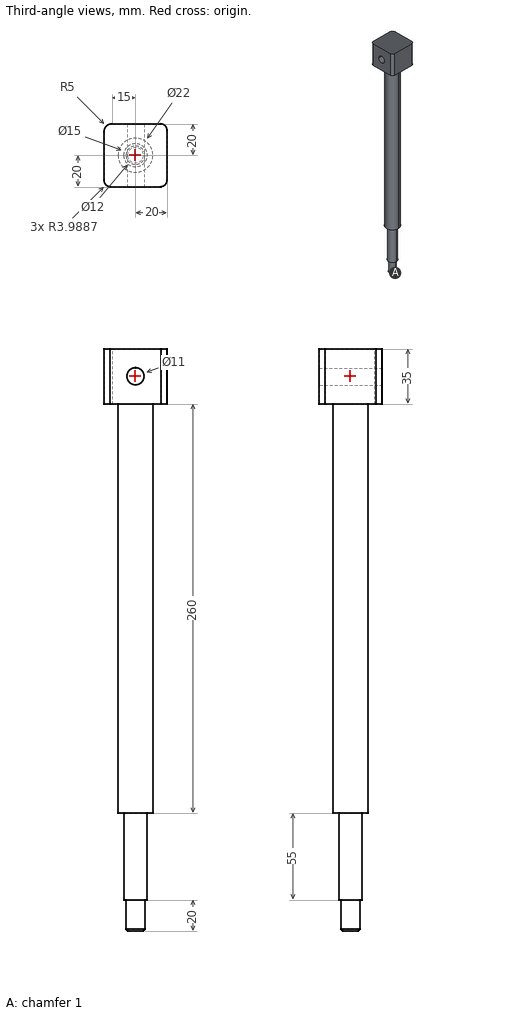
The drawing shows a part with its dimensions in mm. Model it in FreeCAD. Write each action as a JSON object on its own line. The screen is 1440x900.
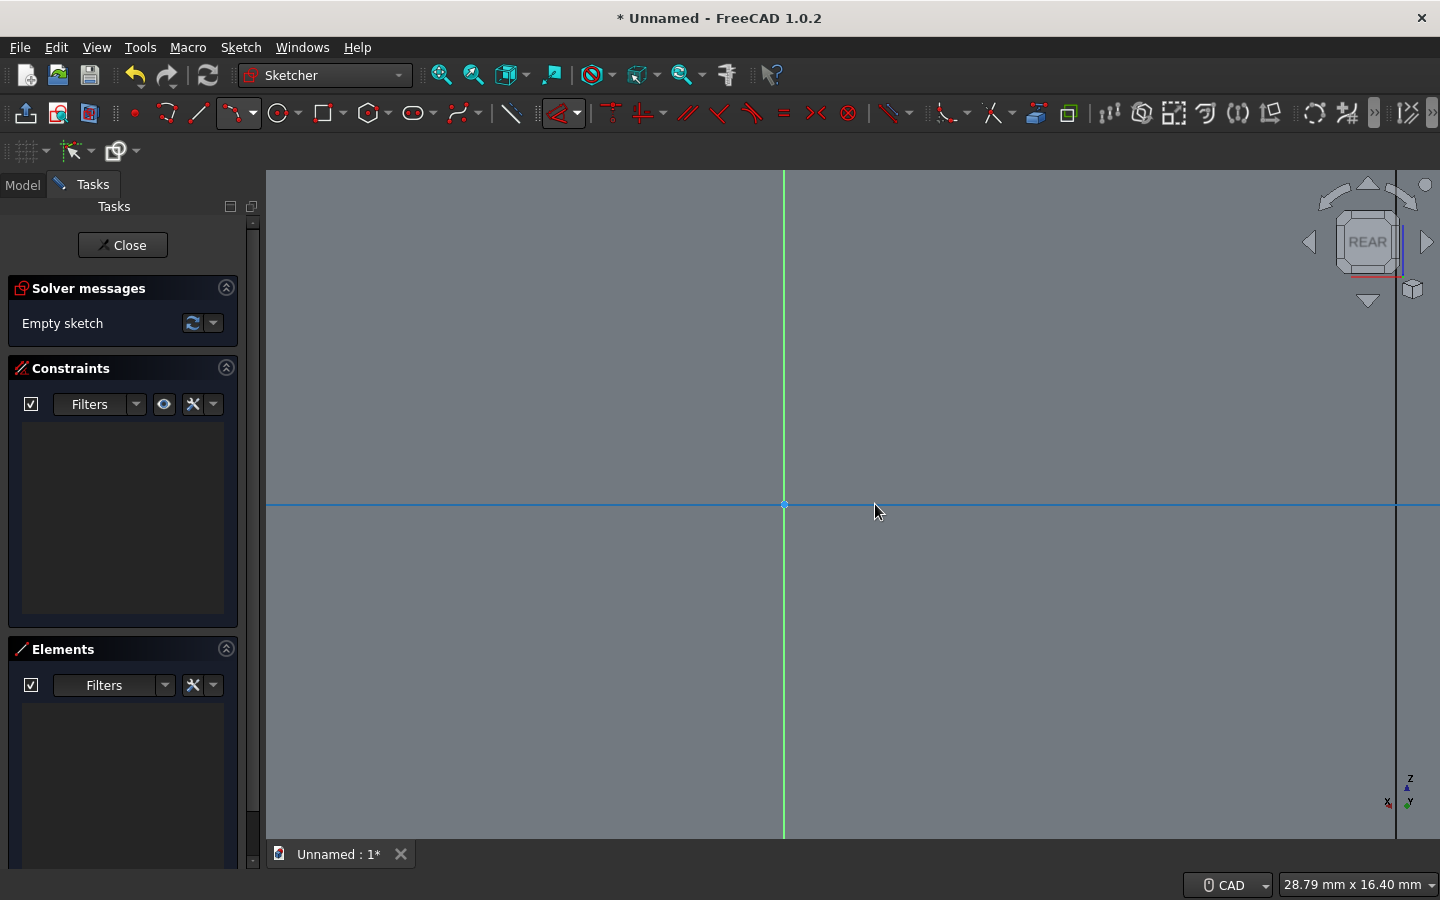
{"action": "left_click", "coordinate": [278, 114]}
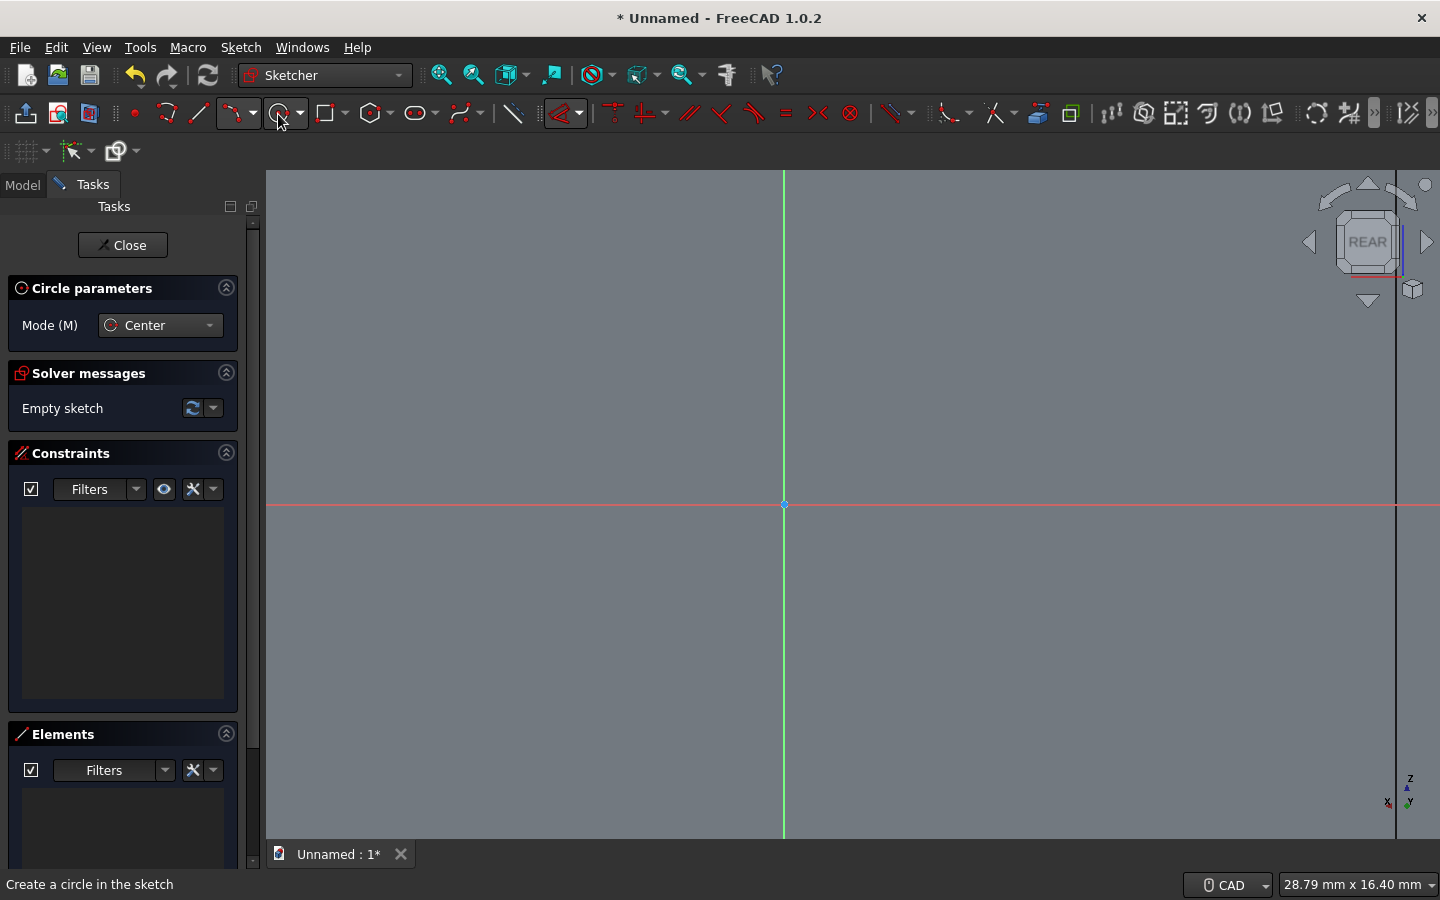
{"action": "left_click", "coordinate": [784, 504]}
{"action": "left_click", "coordinate": [943, 346]}
{"action": "key", "text": "Escape"}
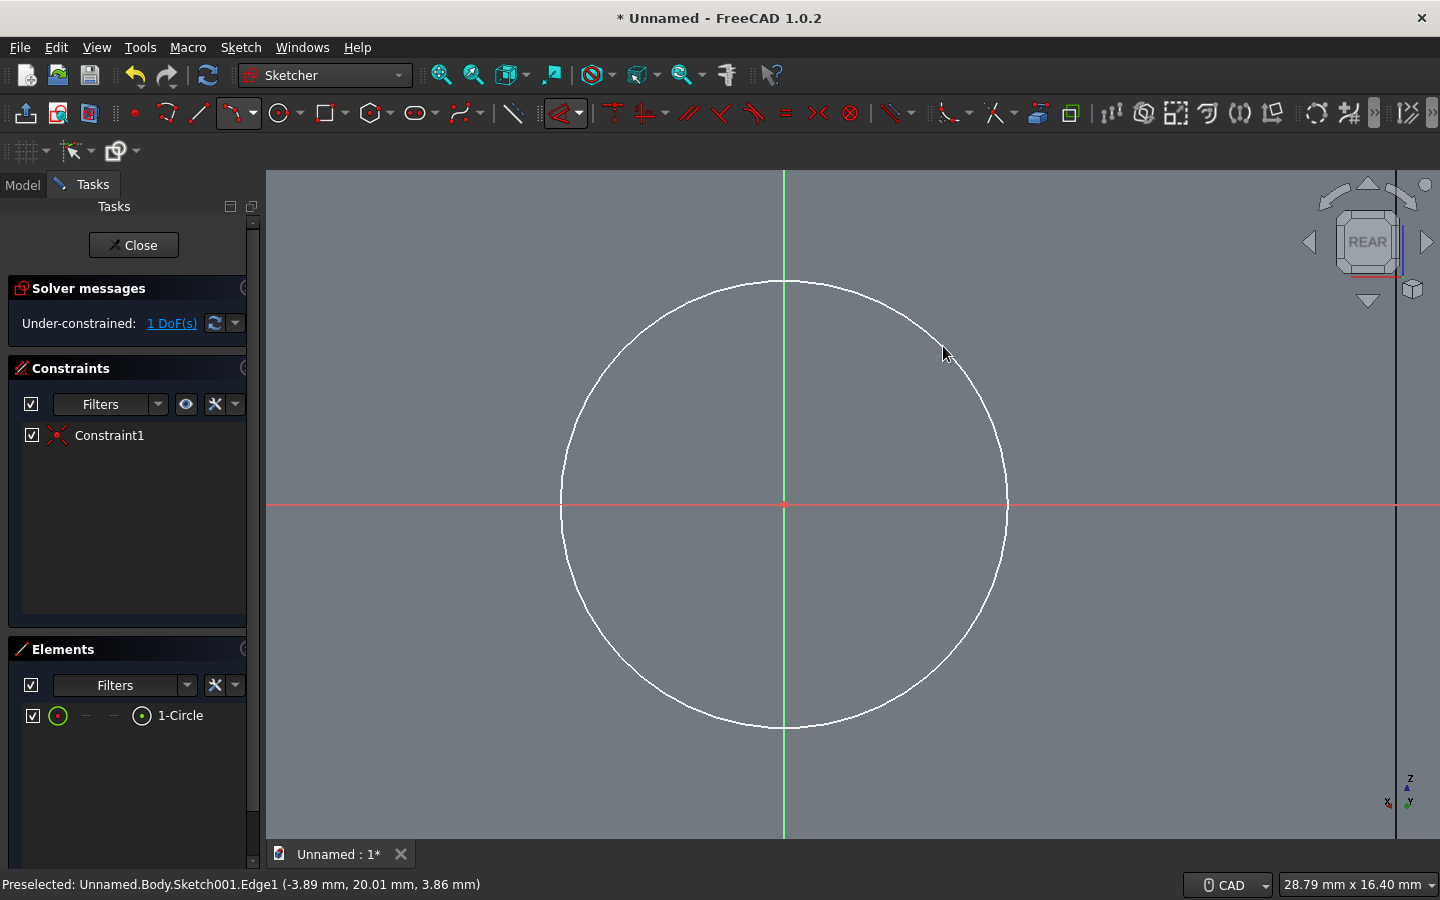
{"action": "left_click", "coordinate": [942, 346]}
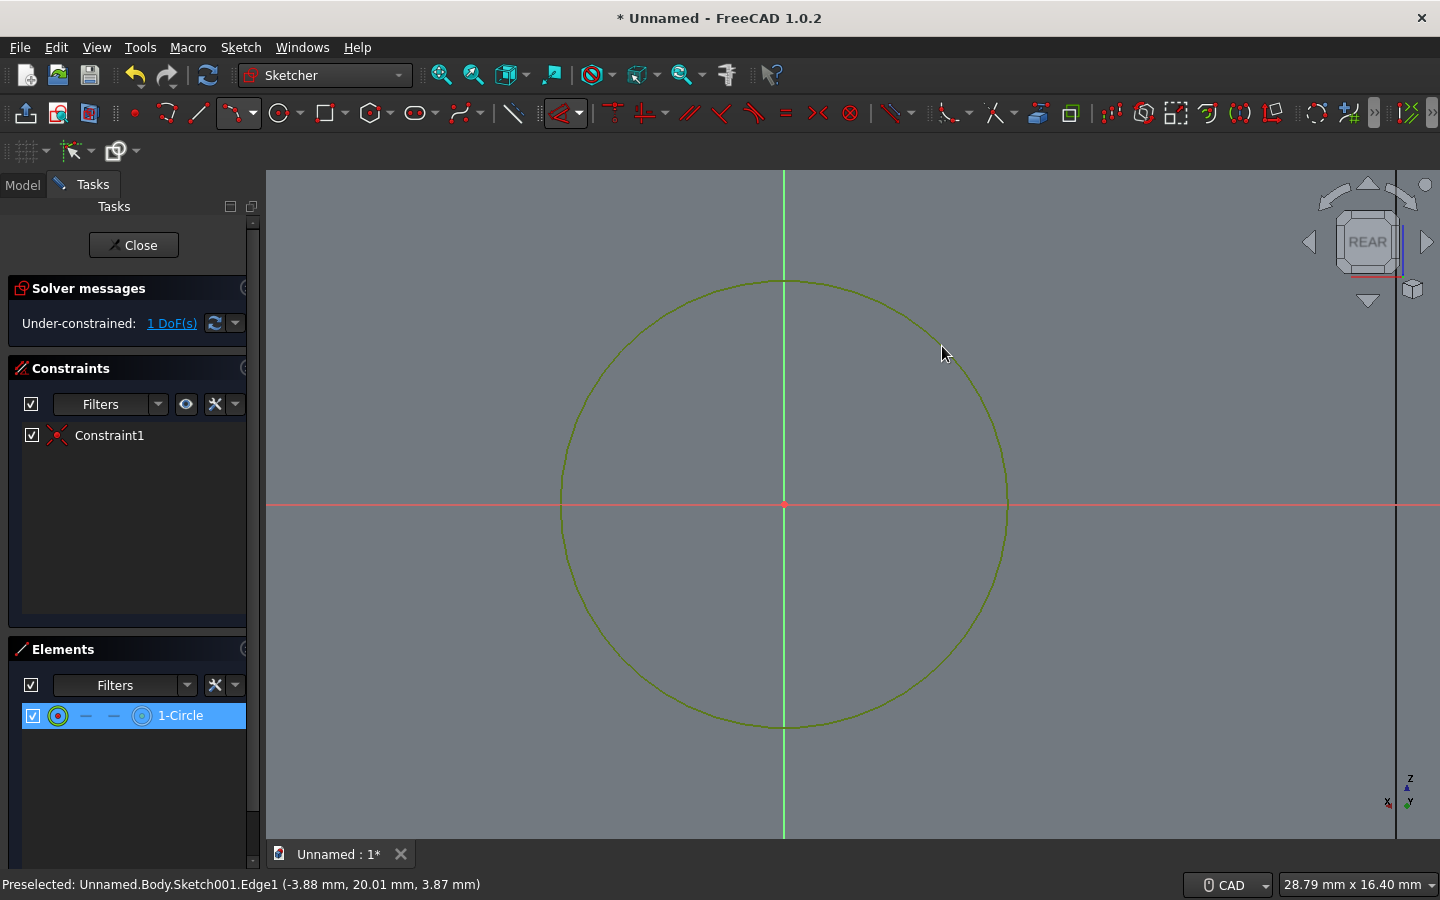
{"action": "left_click", "coordinate": [582, 114]}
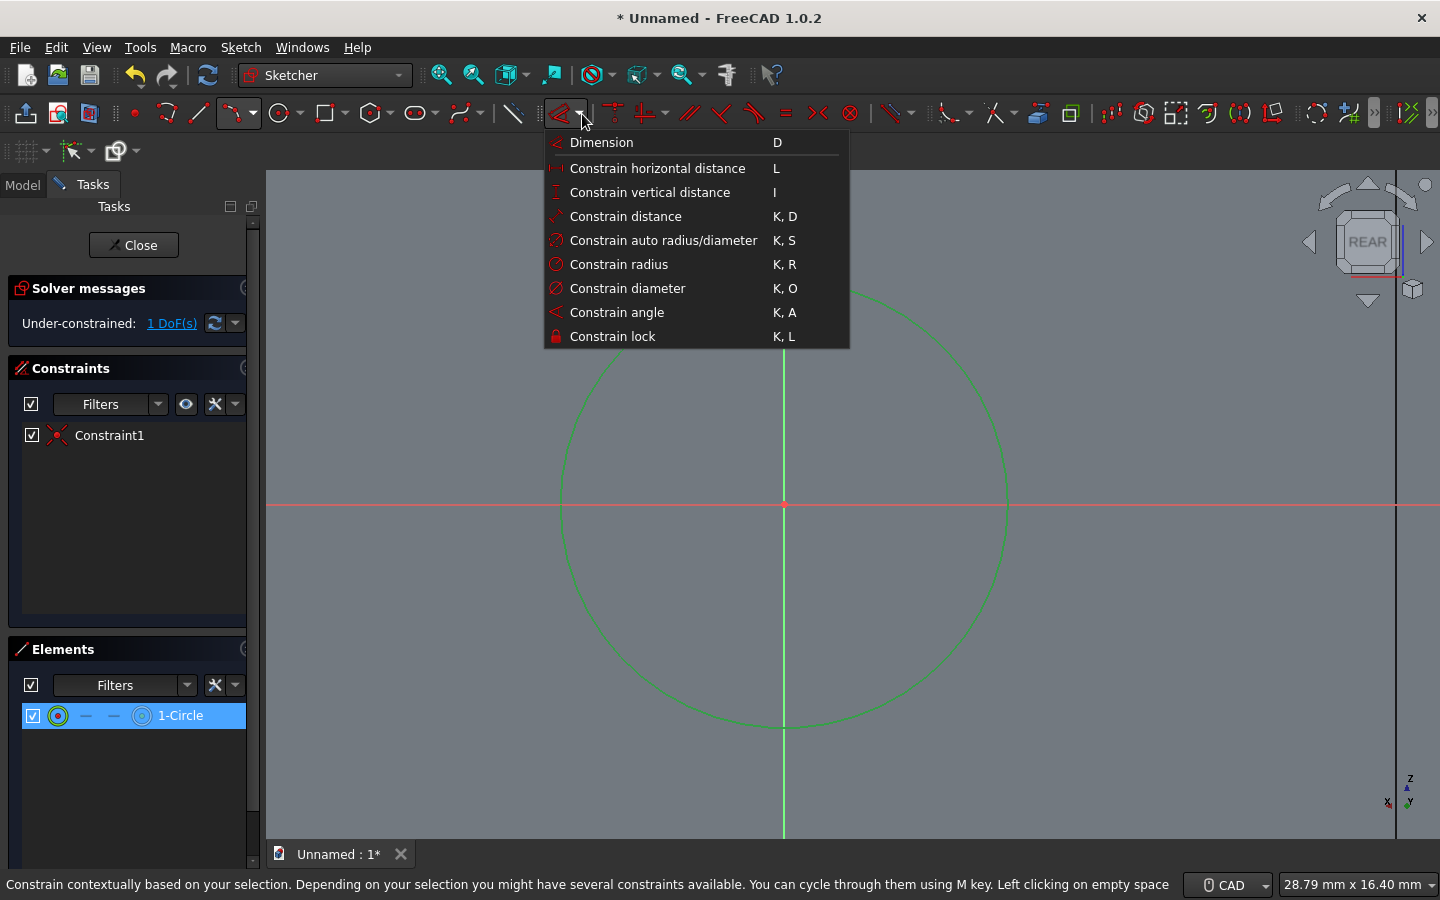
{"action": "left_click", "coordinate": [697, 288]}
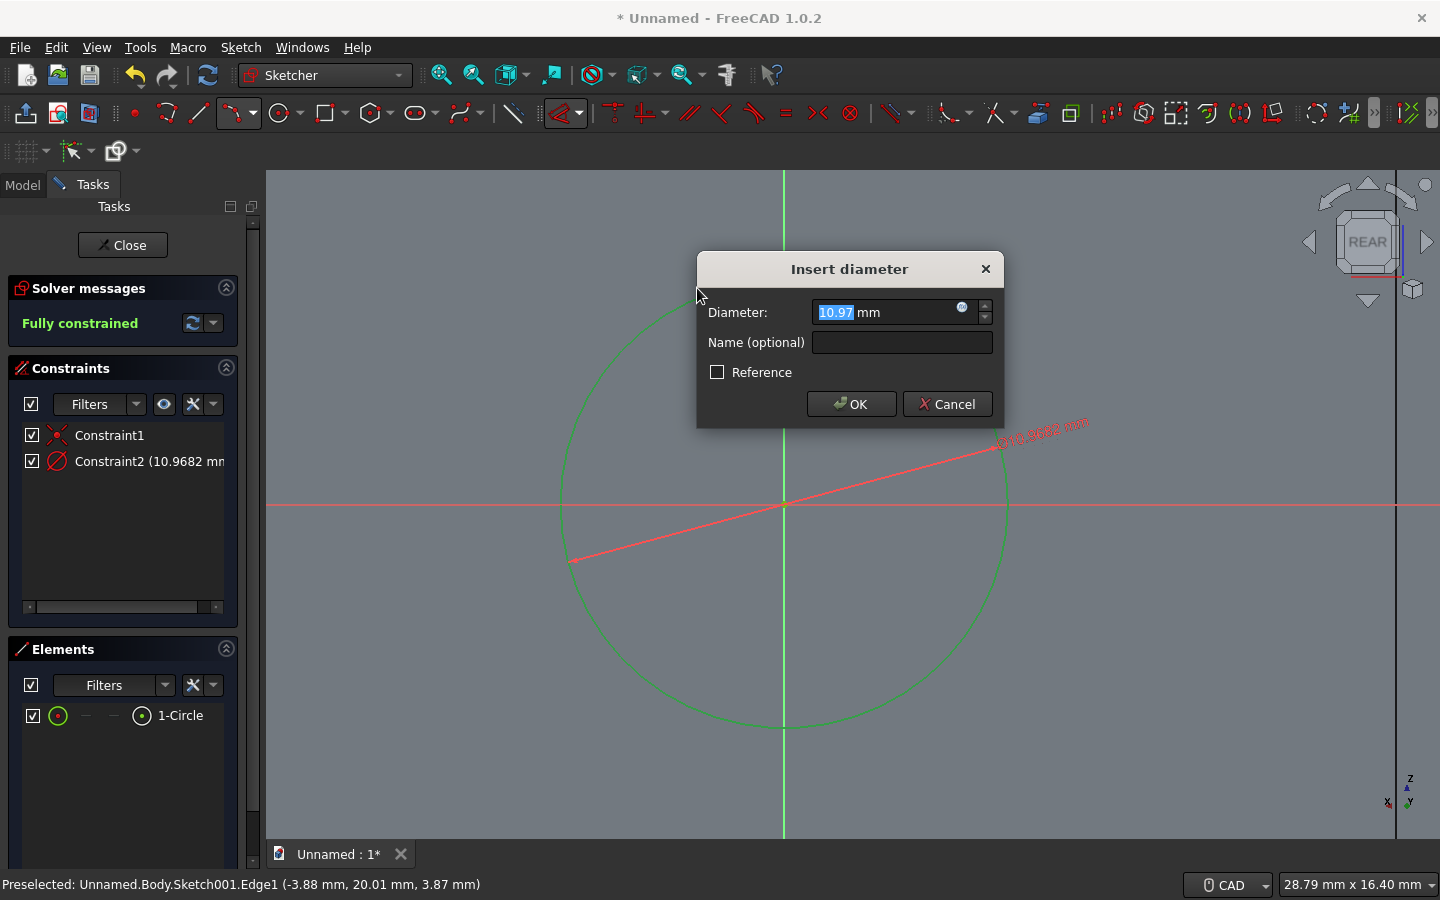
{"action": "type", "text": "11"}
{"action": "key", "text": "Return"}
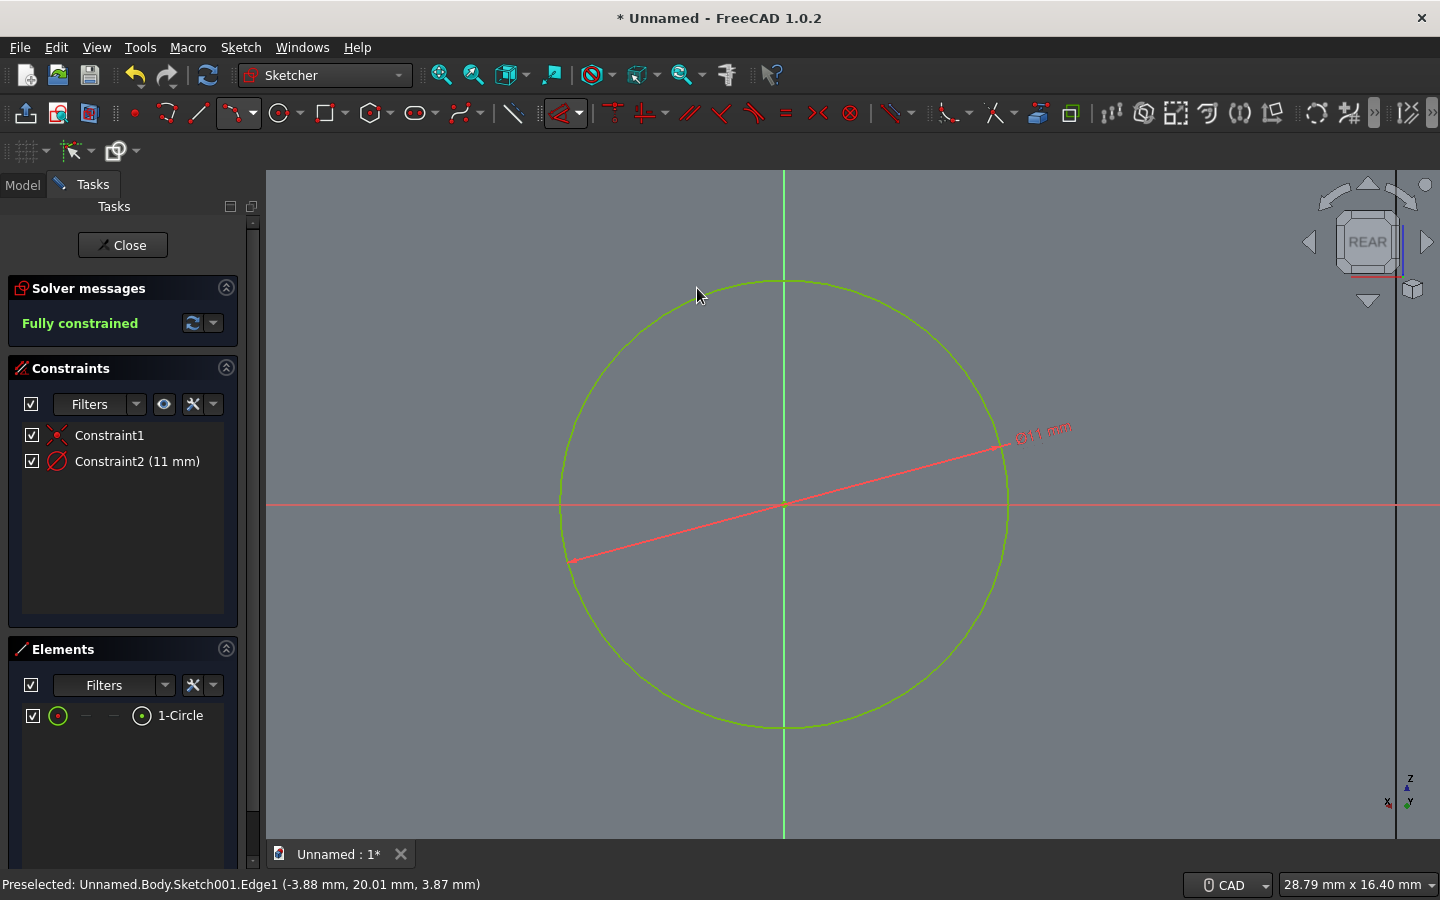
{"action": "left_click", "coordinate": [123, 245]}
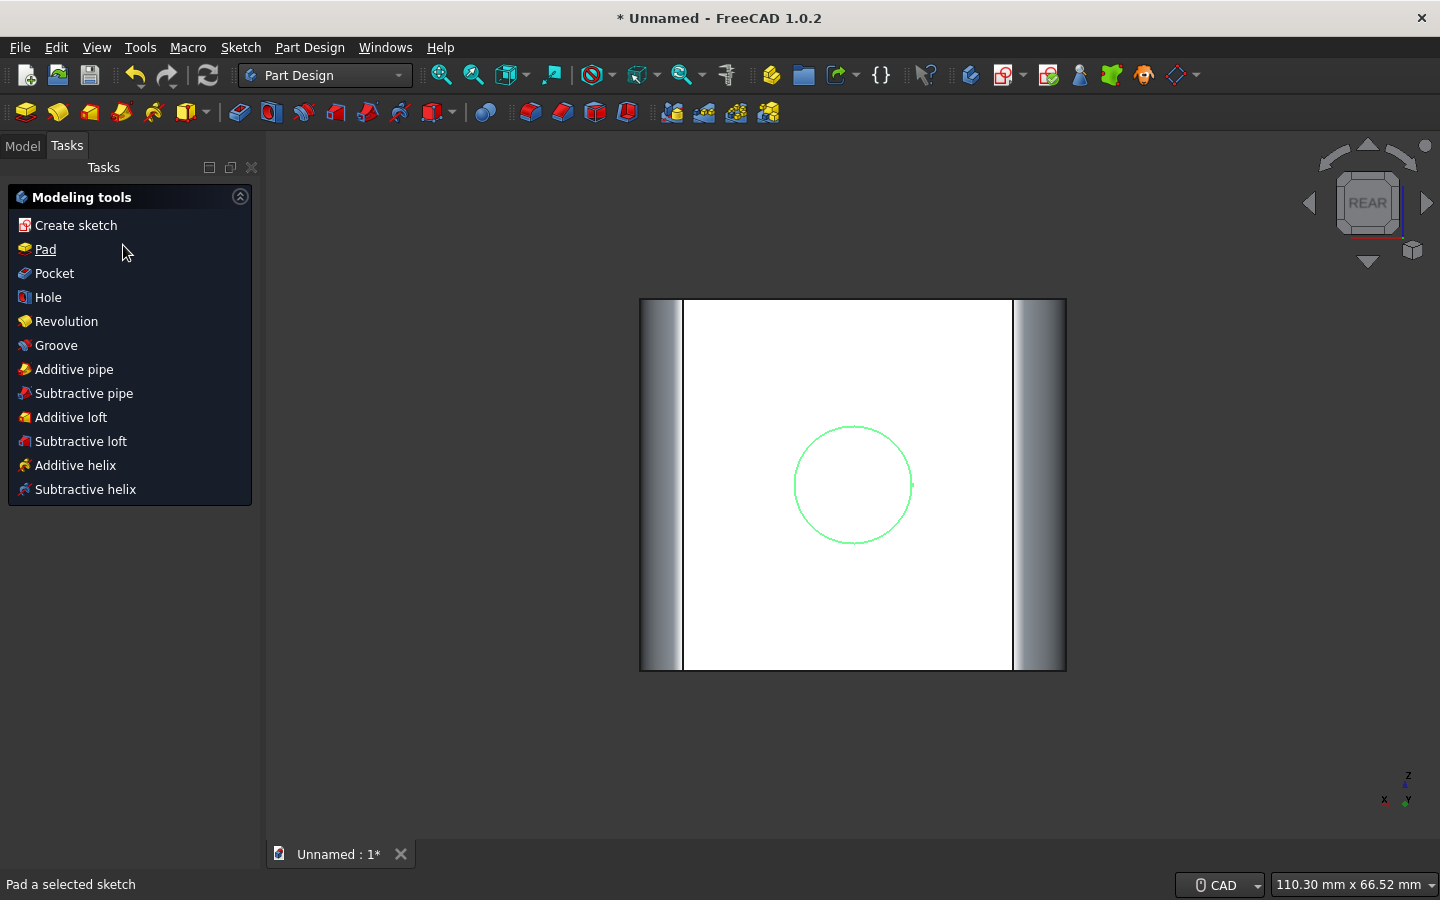
{"action": "left_click", "coordinate": [240, 112]}